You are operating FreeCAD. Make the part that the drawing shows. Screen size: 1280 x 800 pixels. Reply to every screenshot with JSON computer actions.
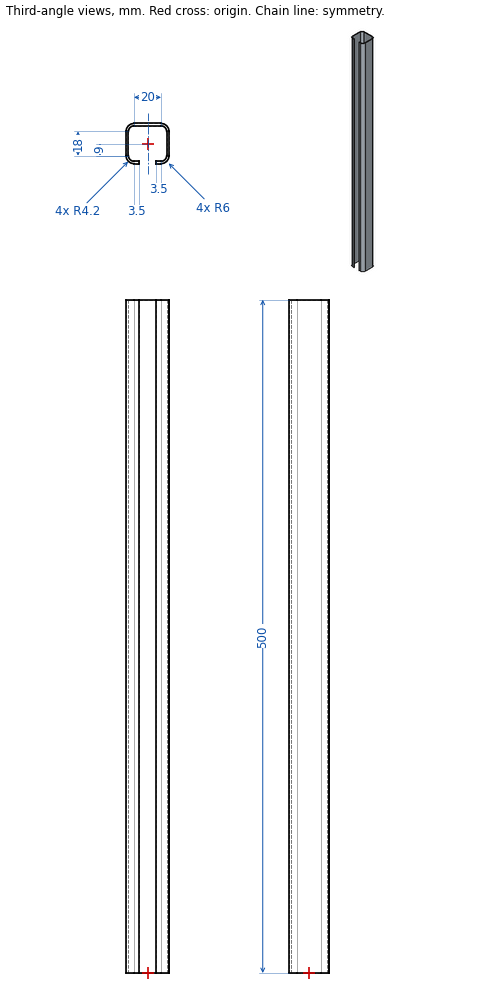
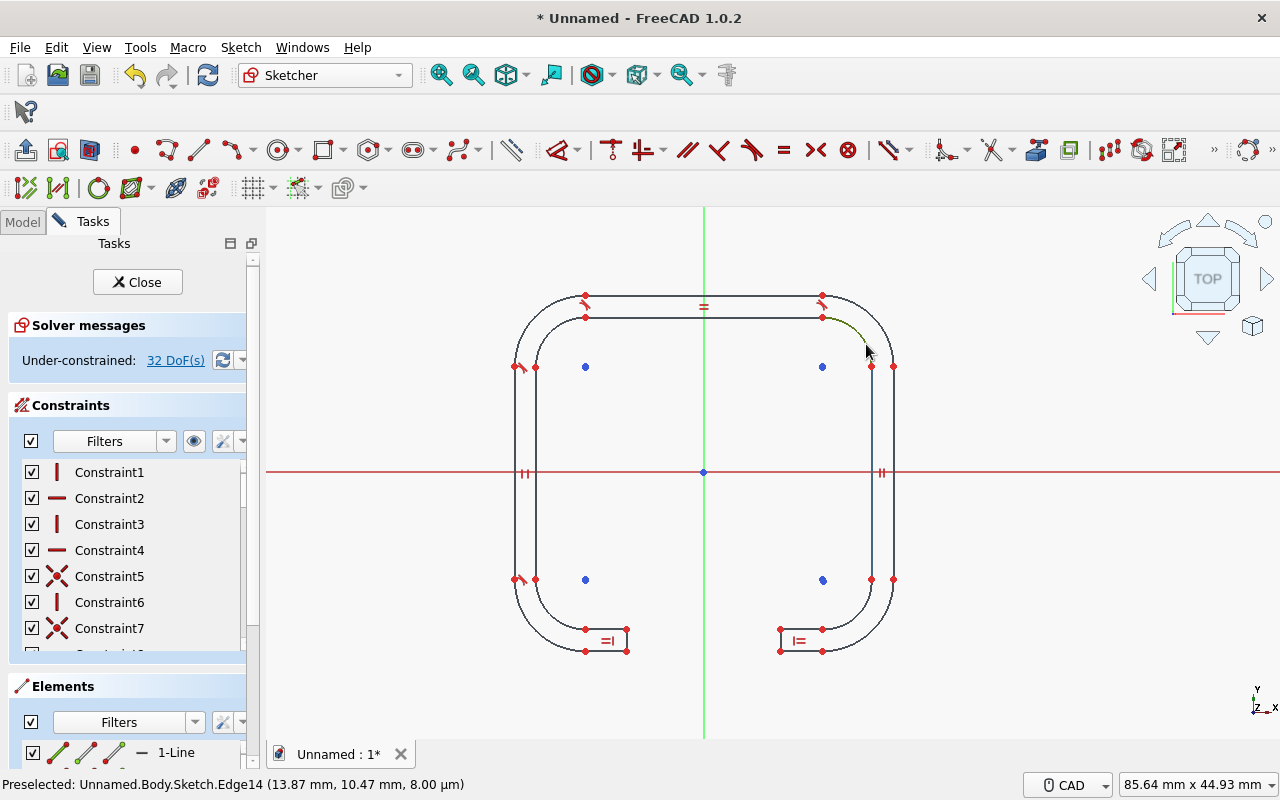
{"action": "left_click", "coordinate": [752, 150]}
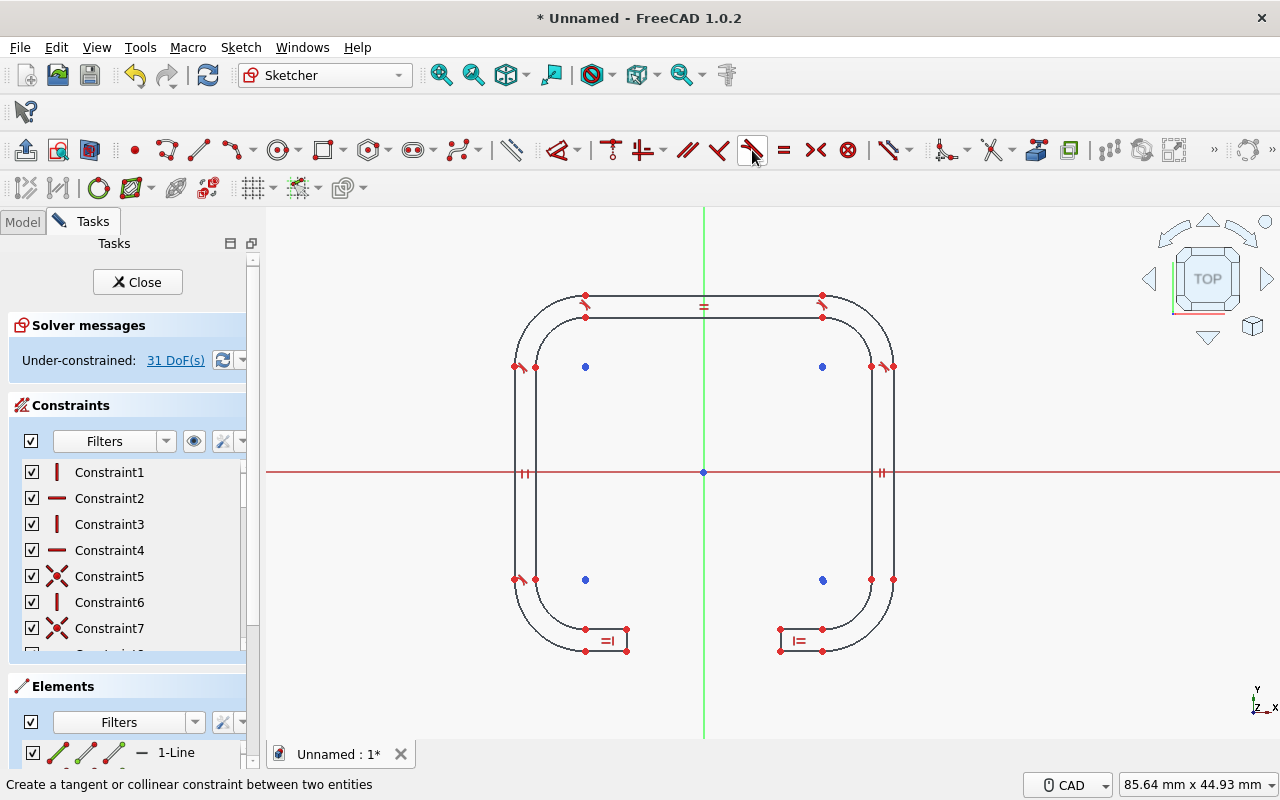
{"action": "left_click", "coordinate": [872, 430]}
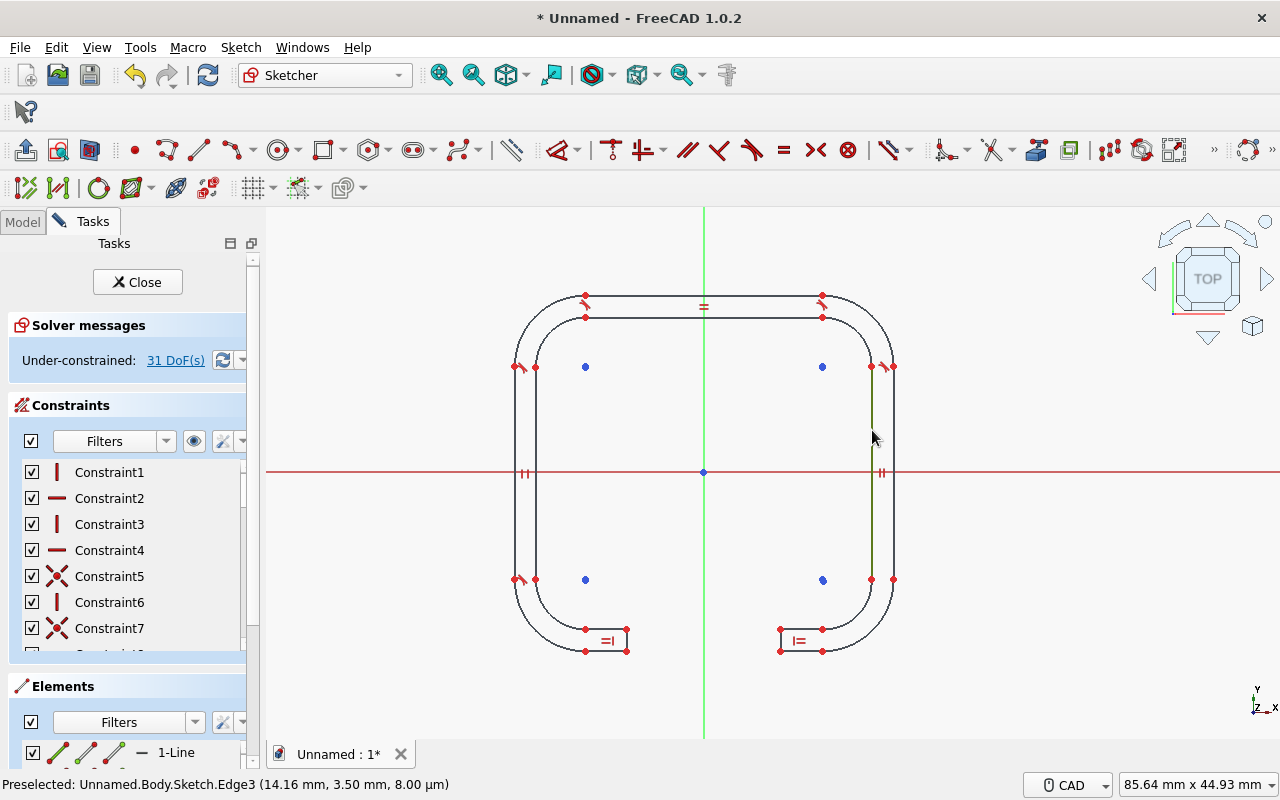
{"action": "left_click", "coordinate": [845, 624]}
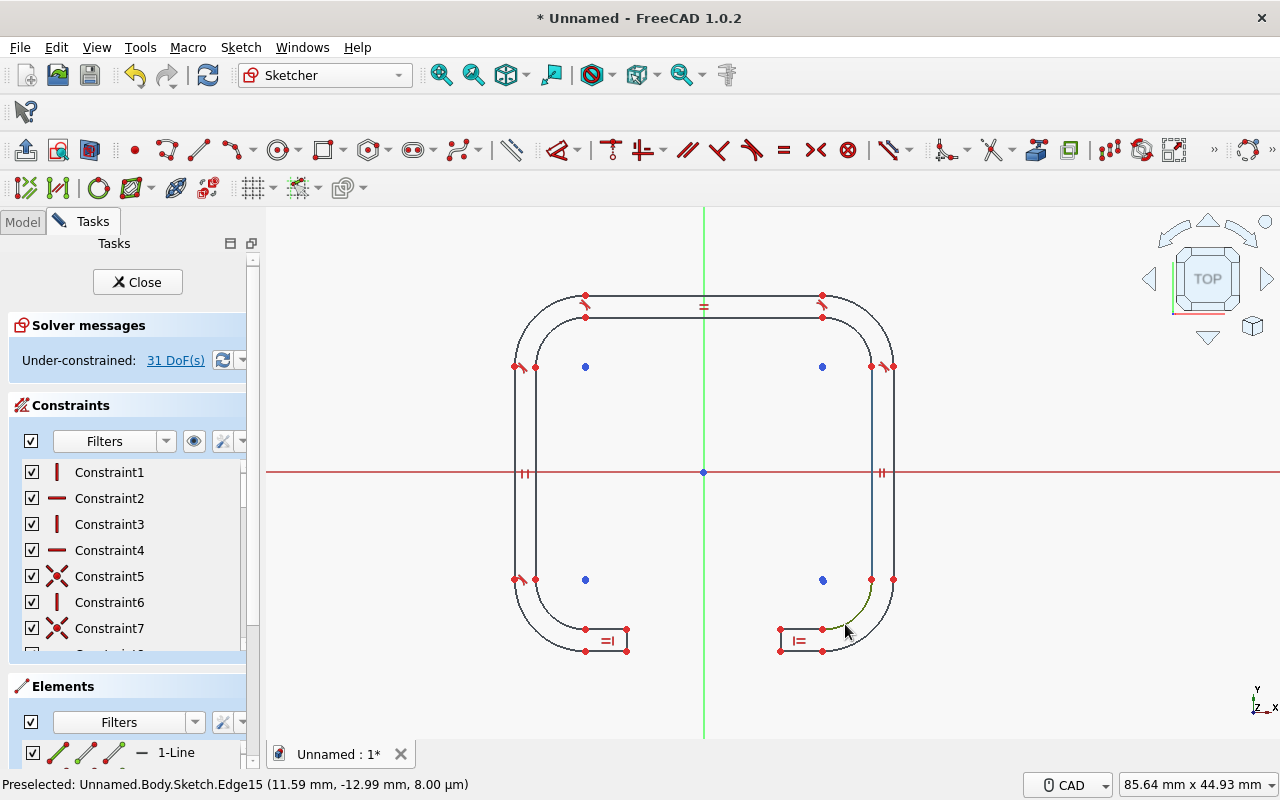
{"action": "left_click", "coordinate": [752, 150]}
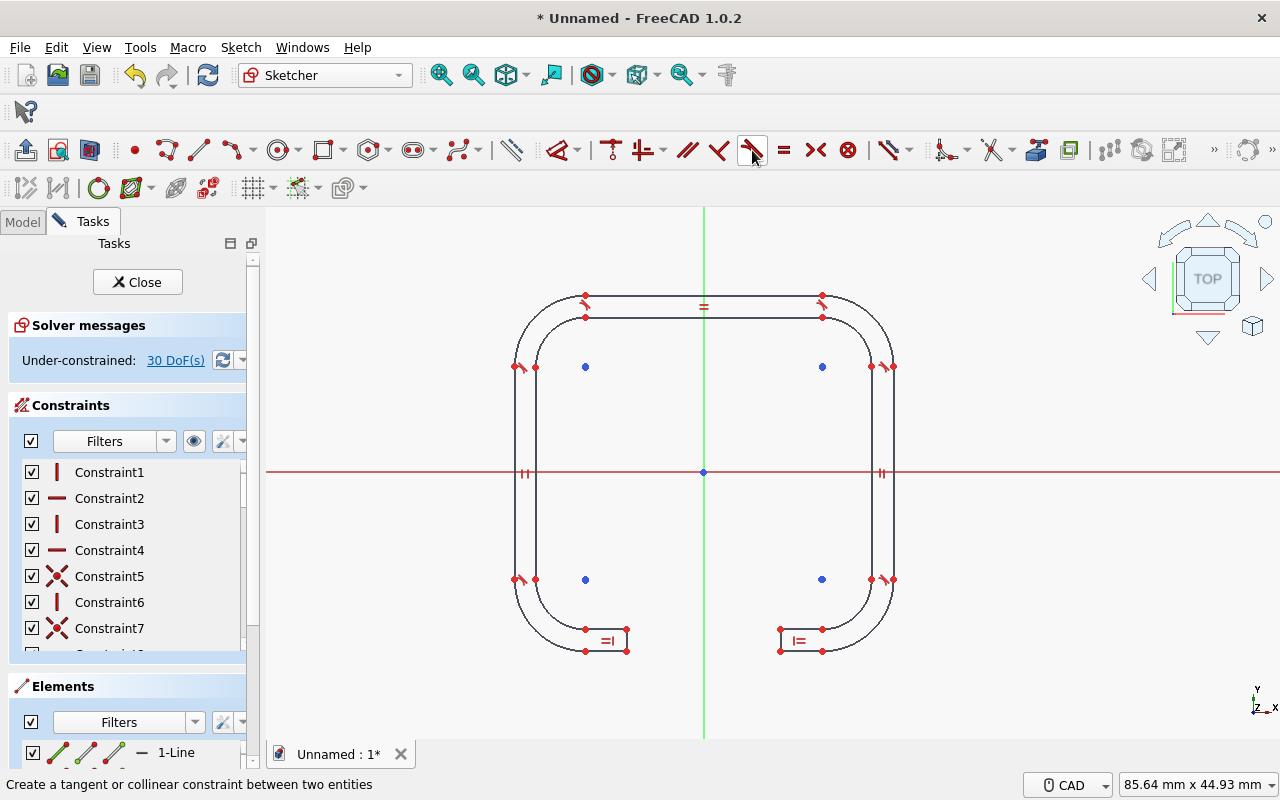
{"action": "left_click", "coordinate": [810, 629]}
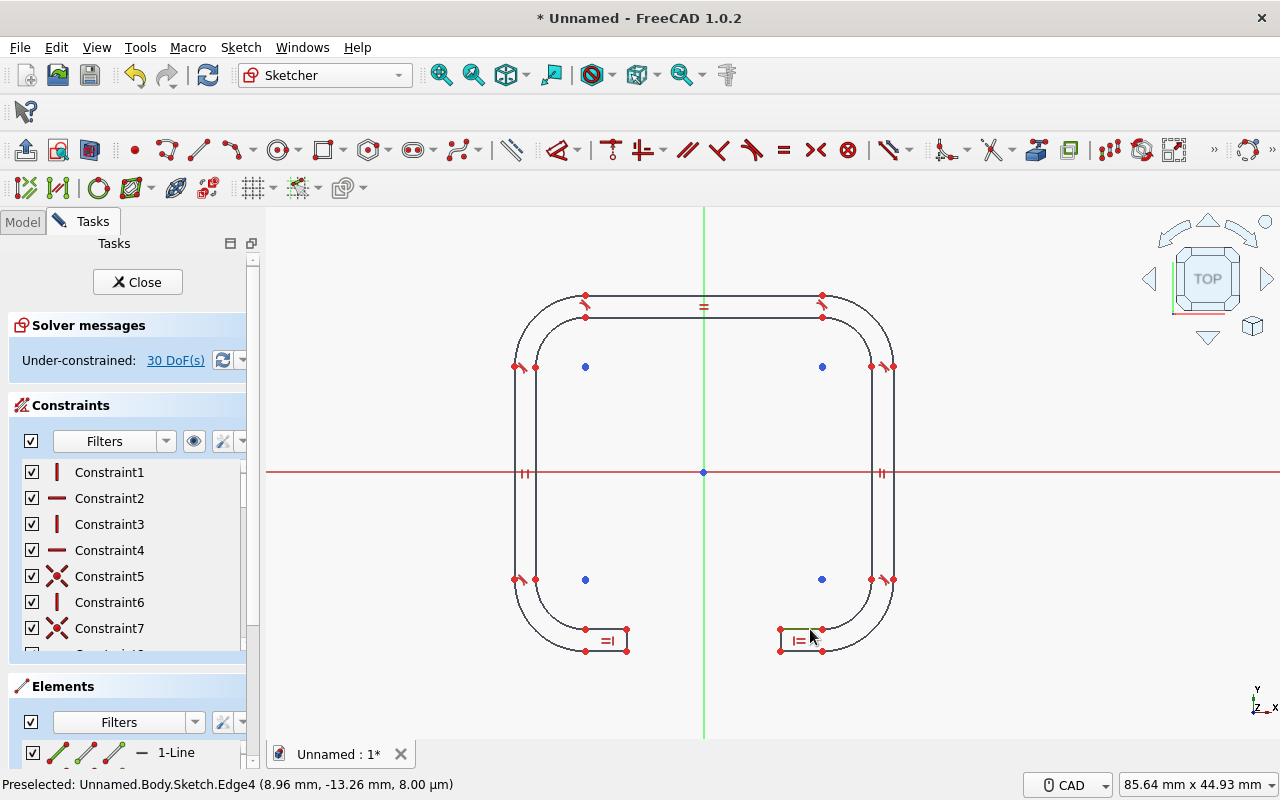
{"action": "left_click", "coordinate": [845, 624]}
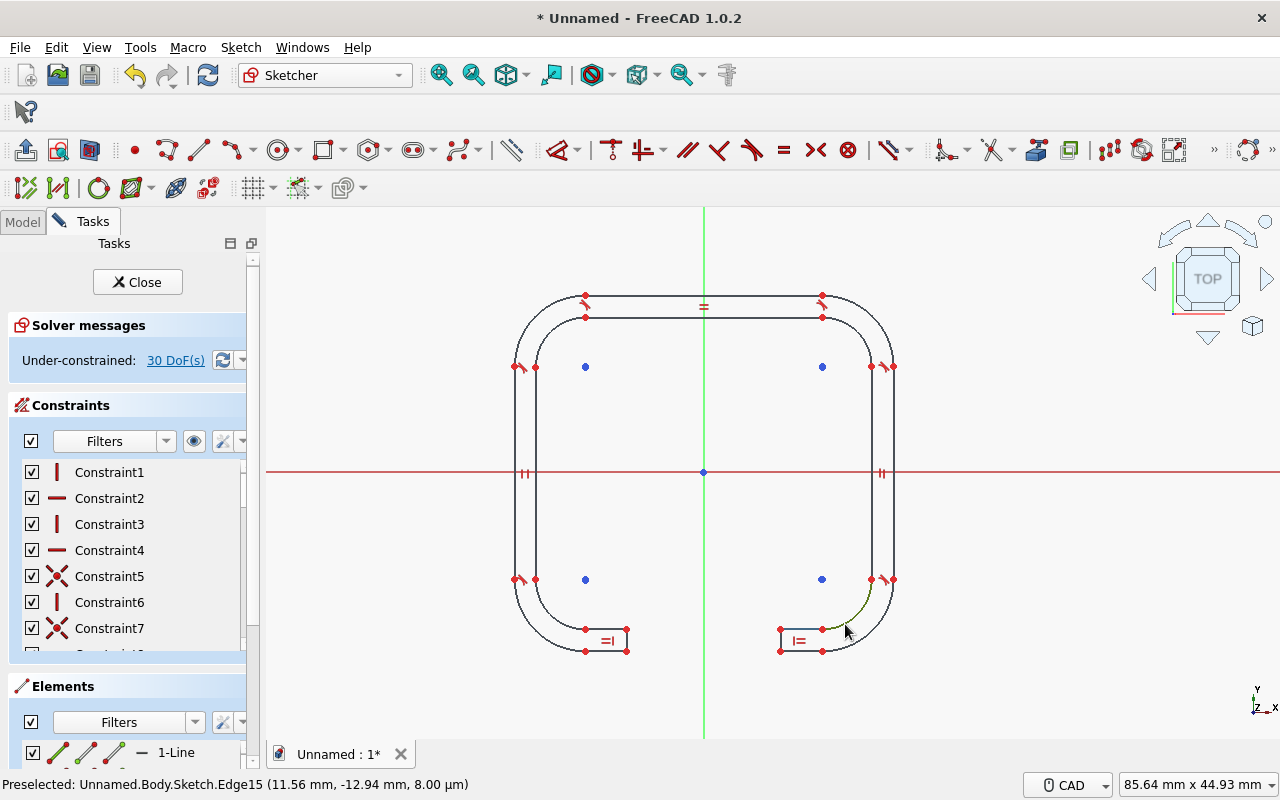
{"action": "left_click", "coordinate": [752, 150]}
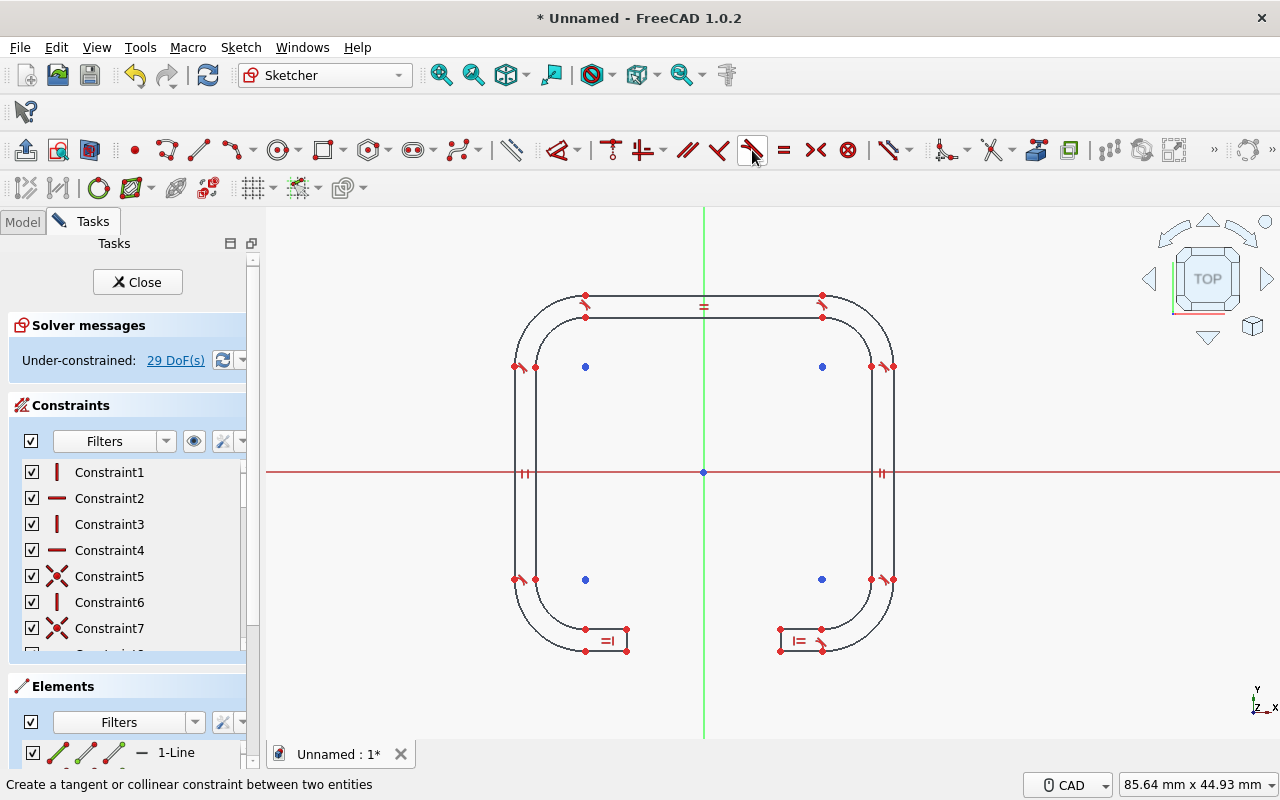
{"action": "left_click", "coordinate": [794, 651]}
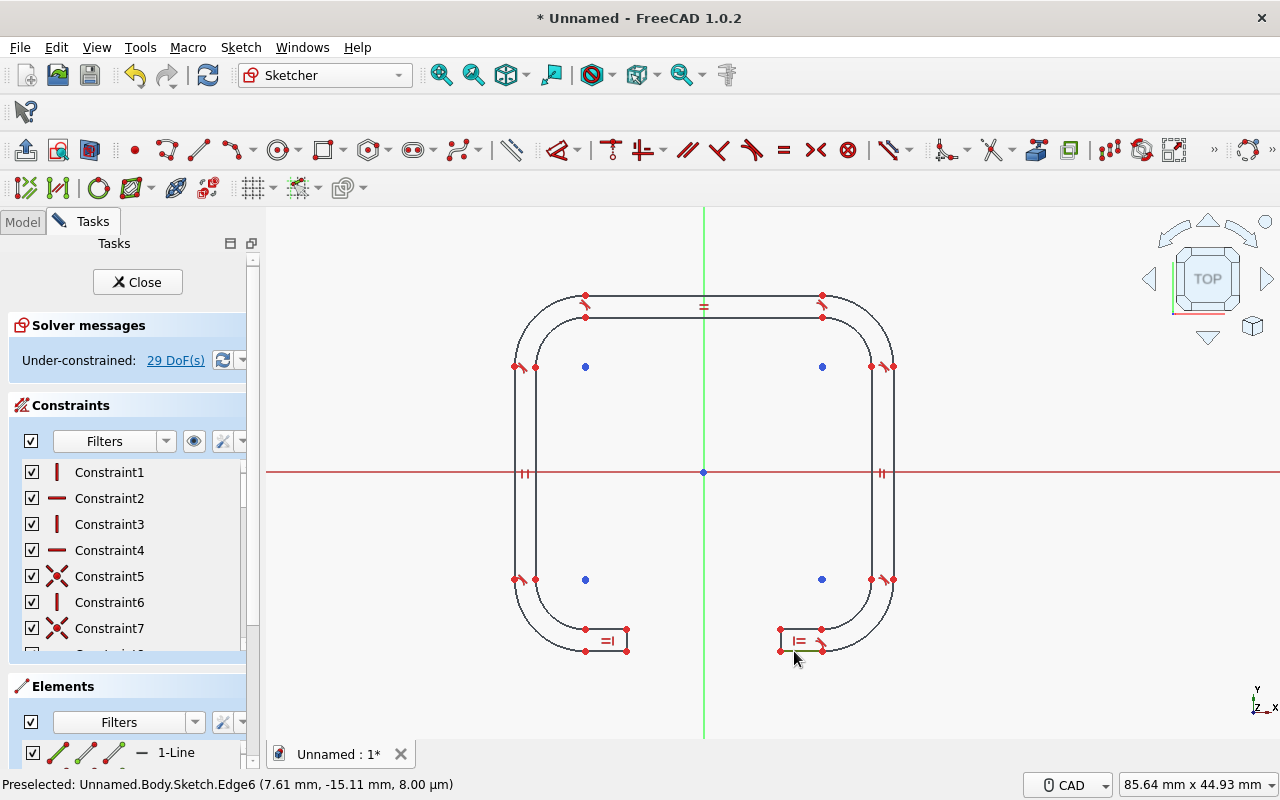
{"action": "left_click", "coordinate": [855, 643]}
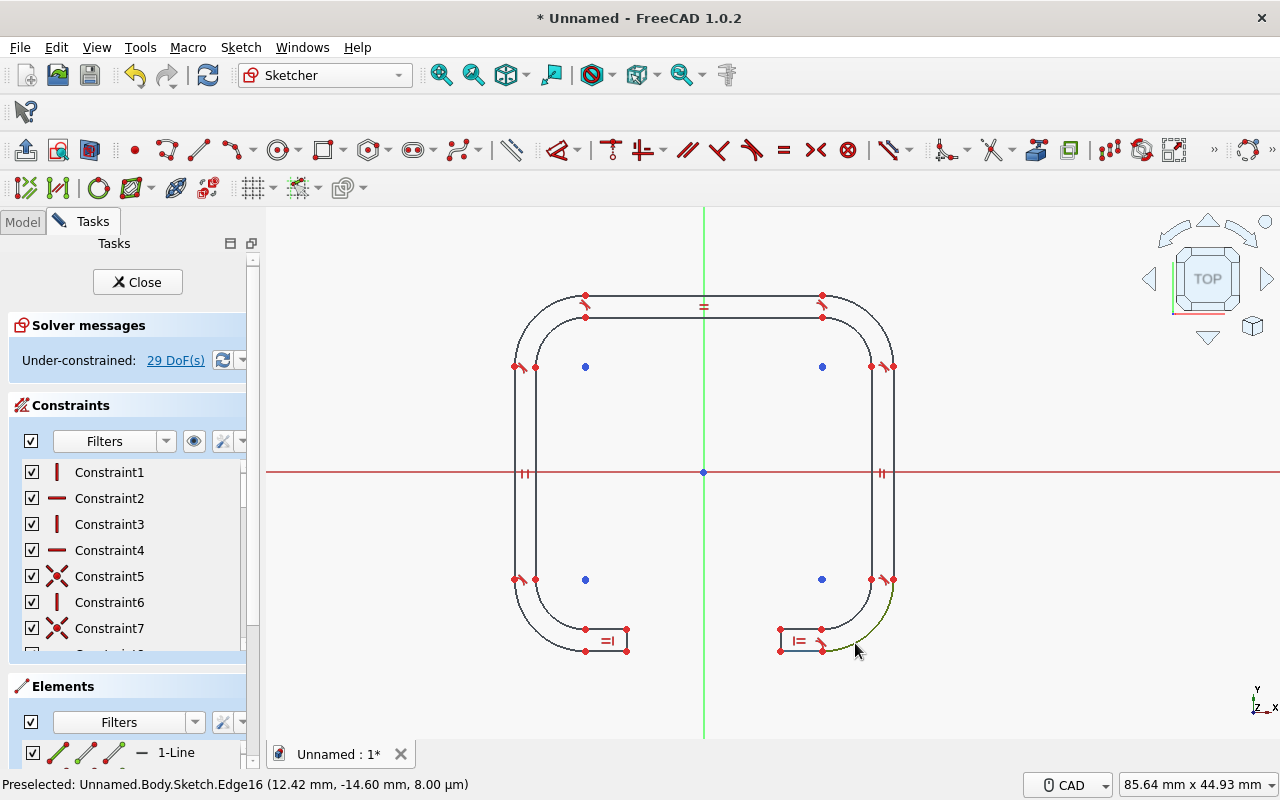
{"action": "left_click", "coordinate": [752, 150]}